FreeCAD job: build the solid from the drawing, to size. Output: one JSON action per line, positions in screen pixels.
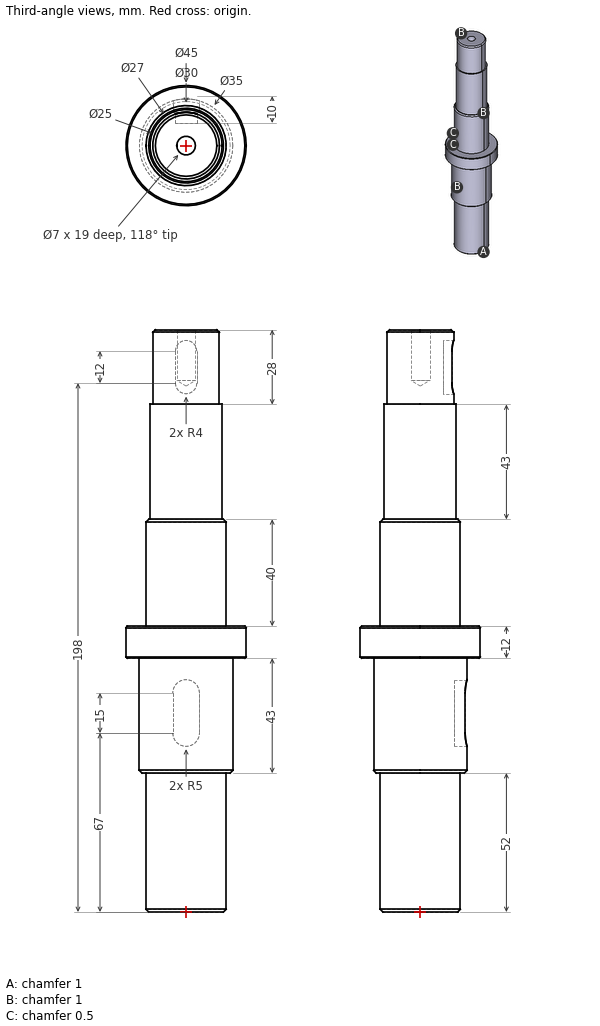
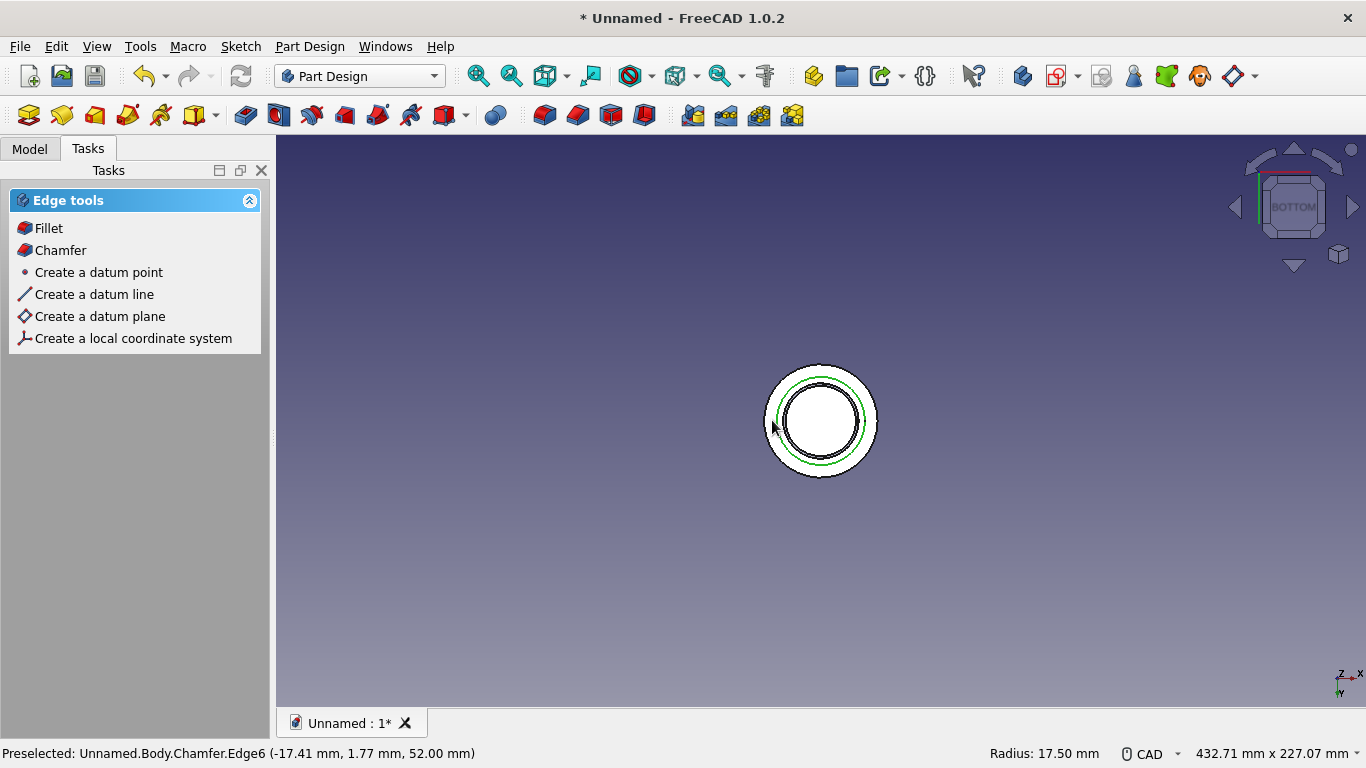
{"action": "key", "text": "0"}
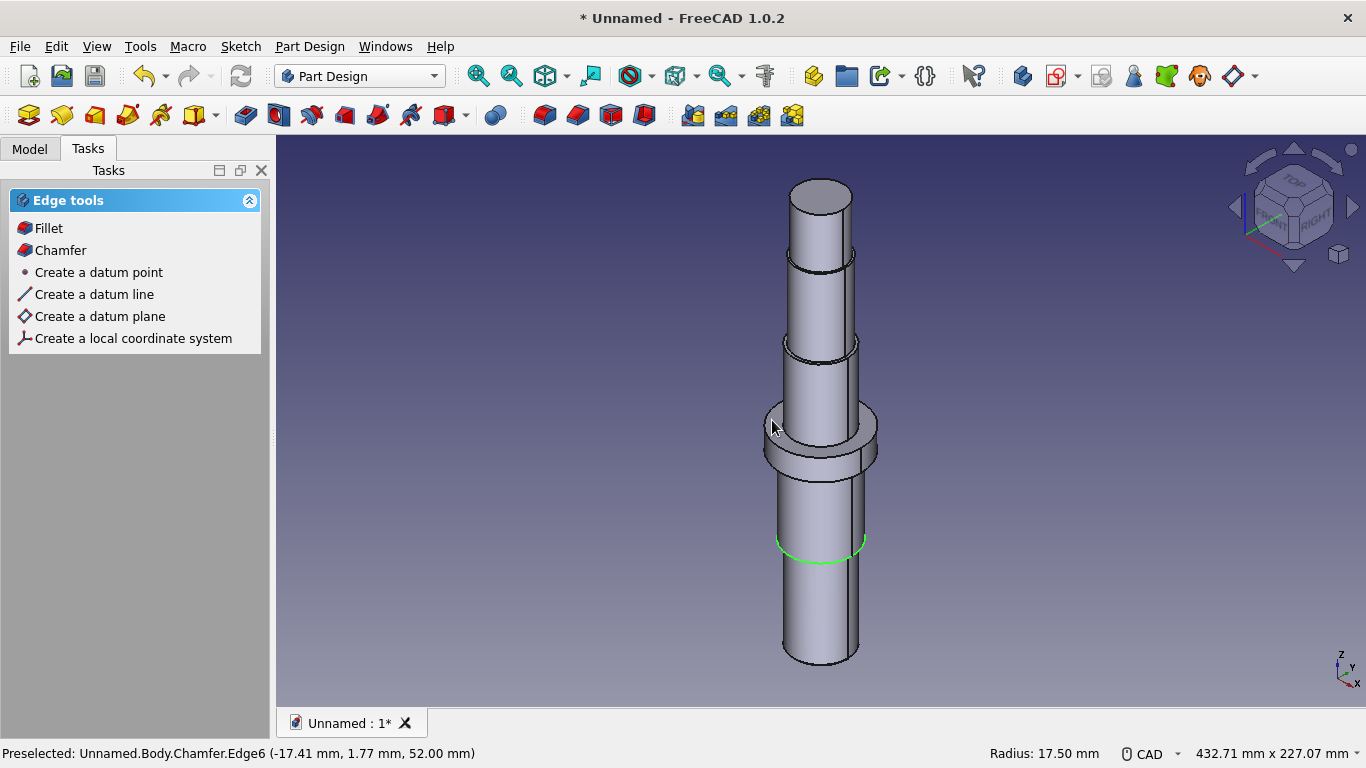
{"action": "left_click", "coordinate": [787, 352], "text": "ctrl"}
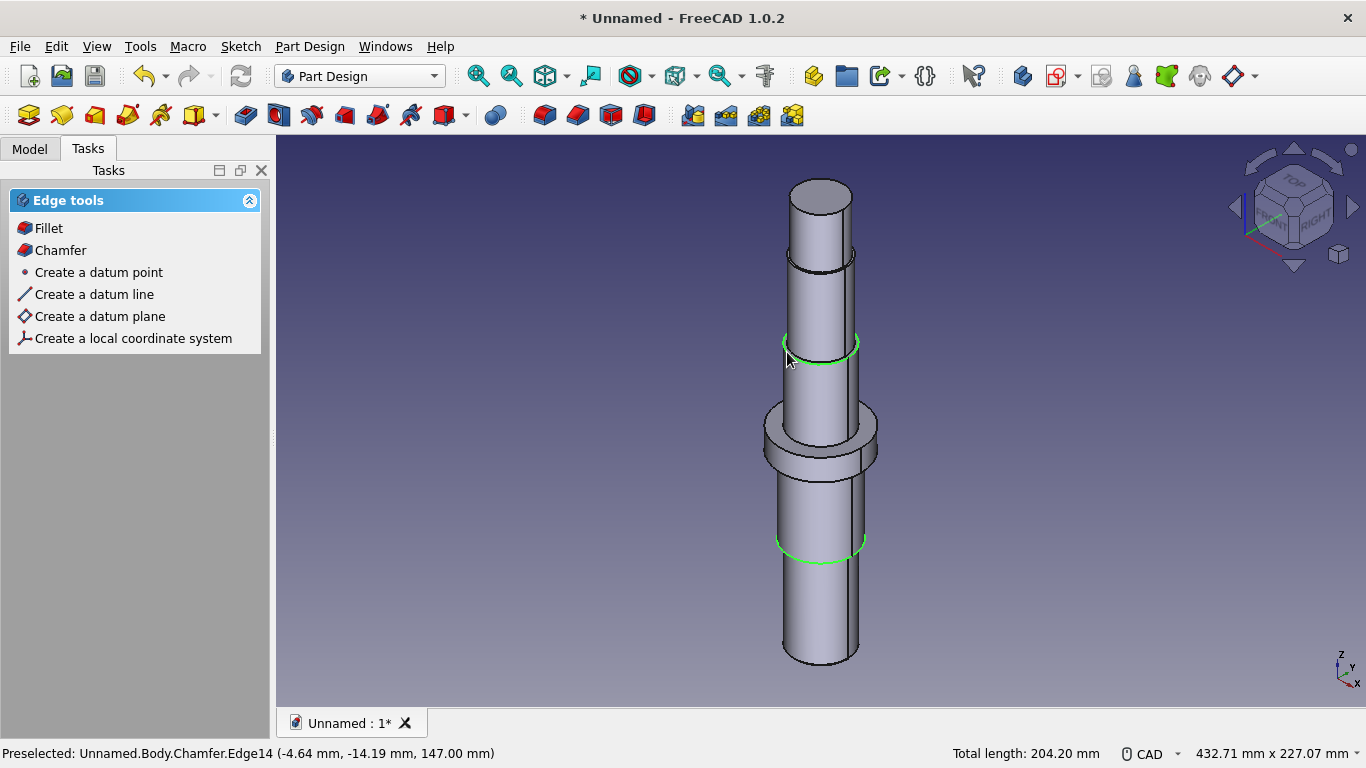
{"action": "left_click", "coordinate": [790, 193], "text": "ctrl"}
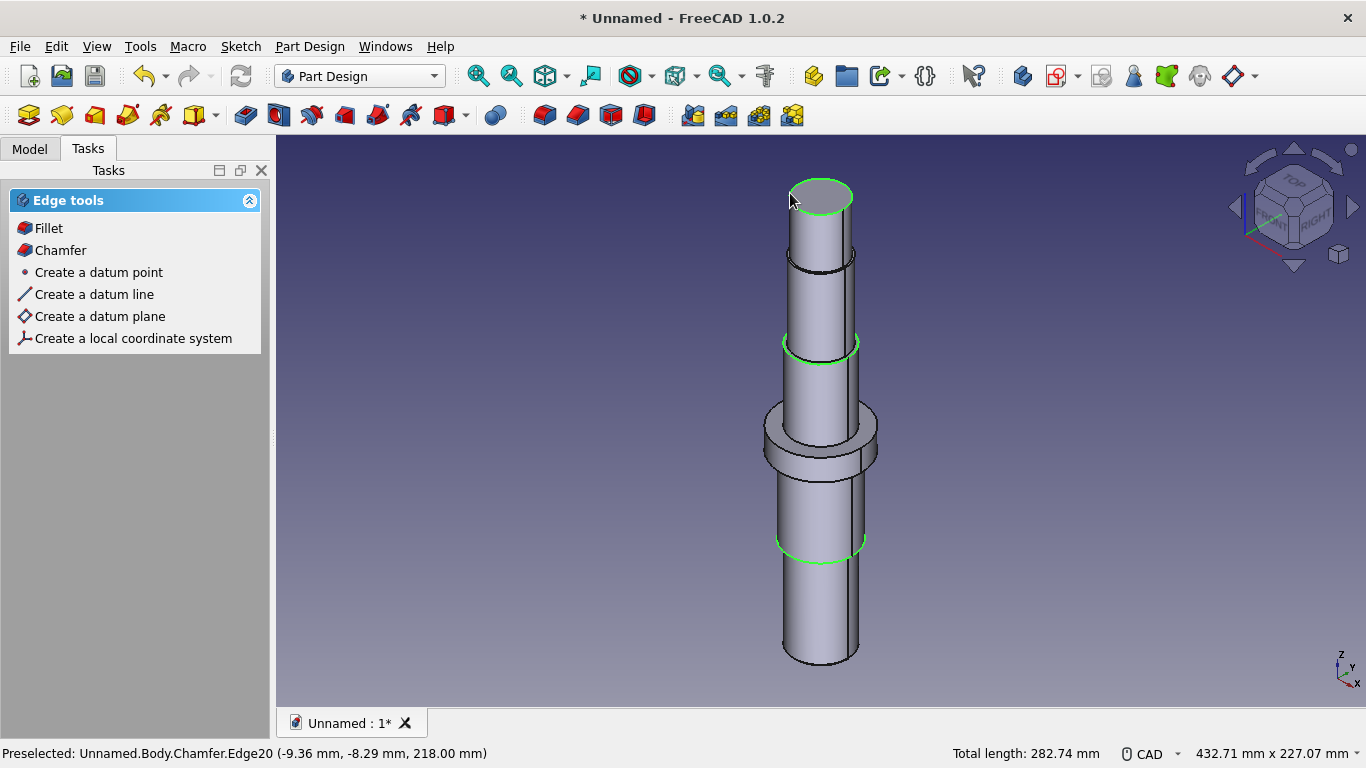
{"action": "left_click", "coordinate": [578, 116]}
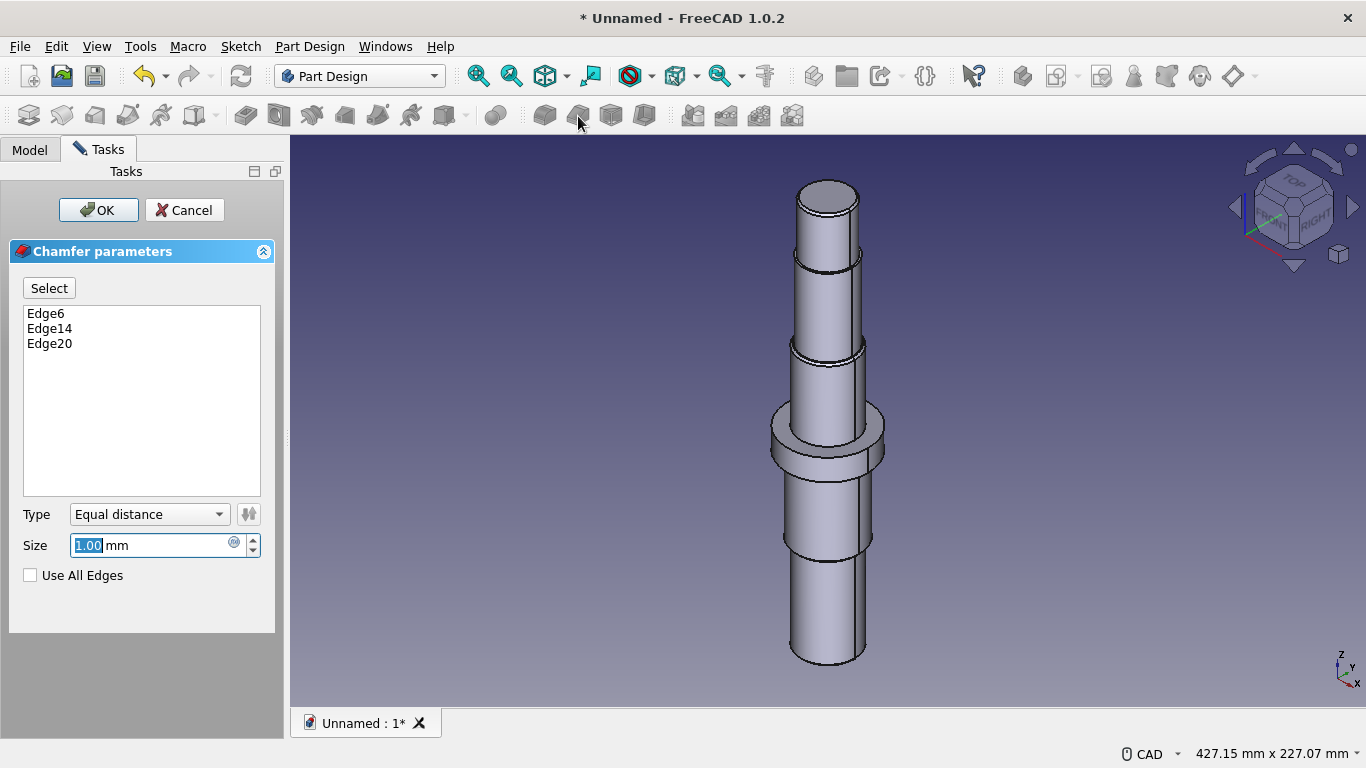
{"action": "type", "text": "1"}
{"action": "key", "text": "Tab"}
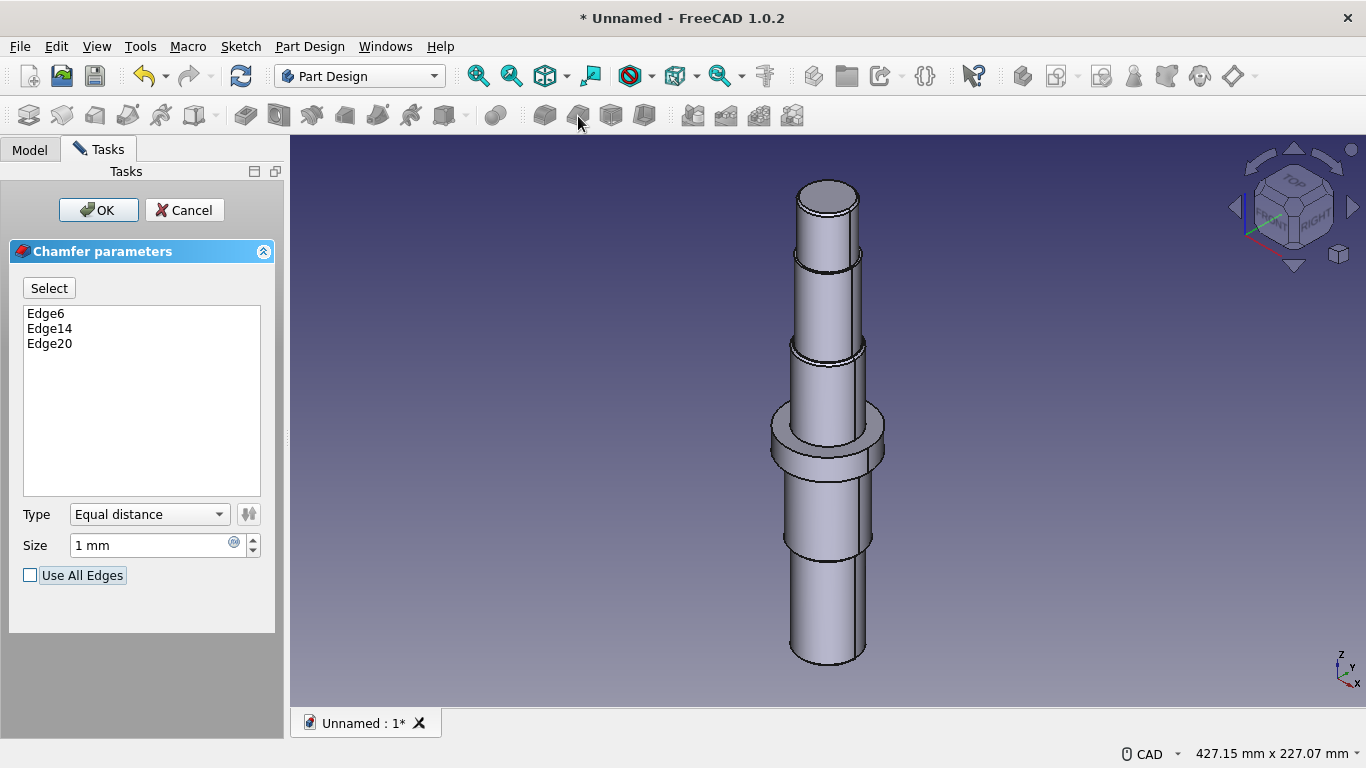
{"action": "left_click", "coordinate": [99, 210]}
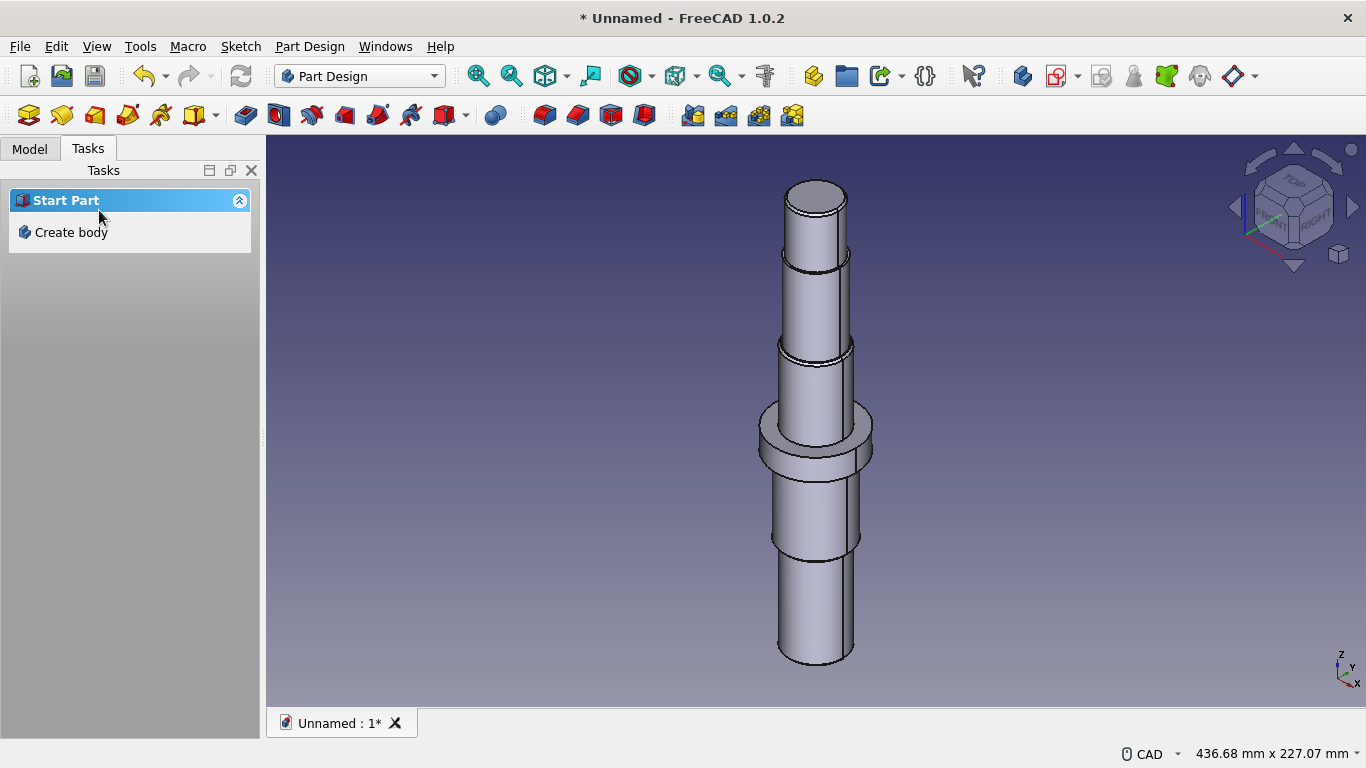
{"action": "left_click", "coordinate": [765, 464]}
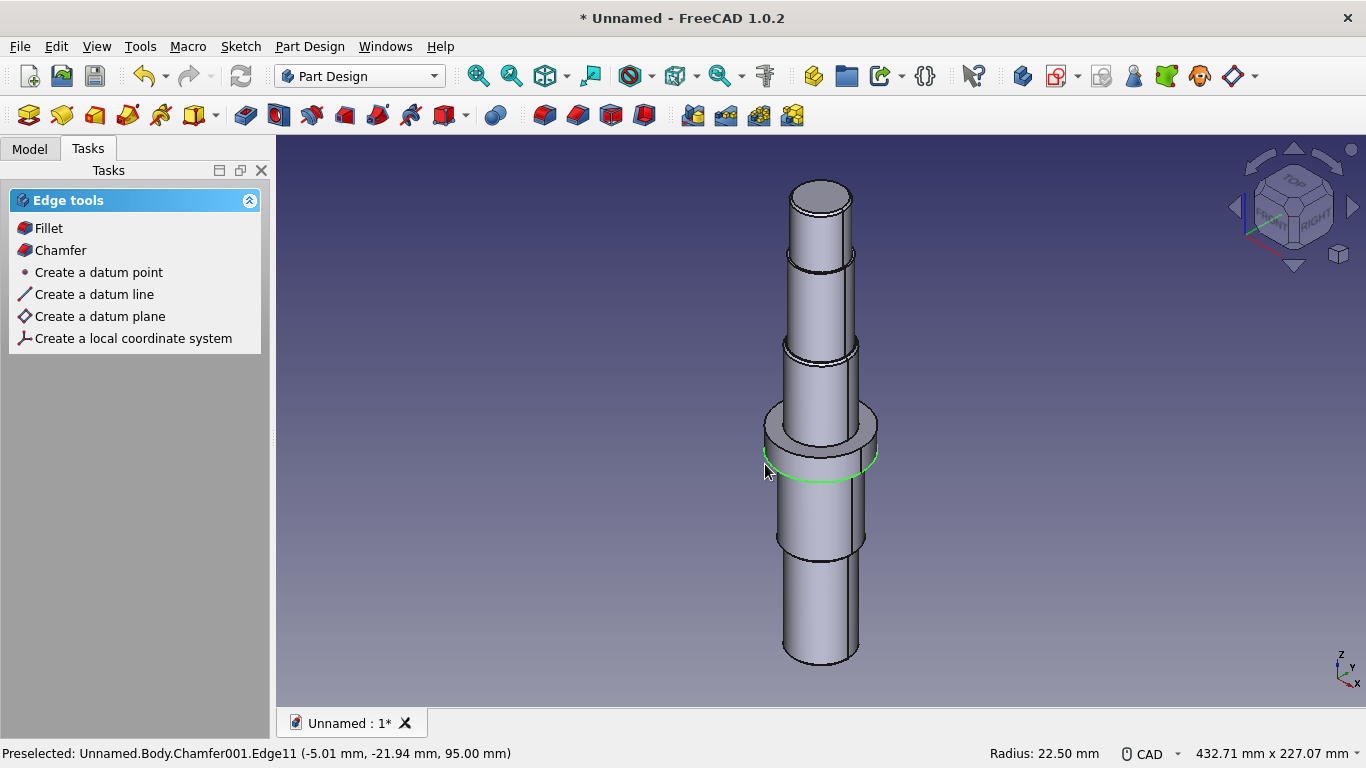
{"action": "left_click", "coordinate": [770, 439], "text": "ctrl"}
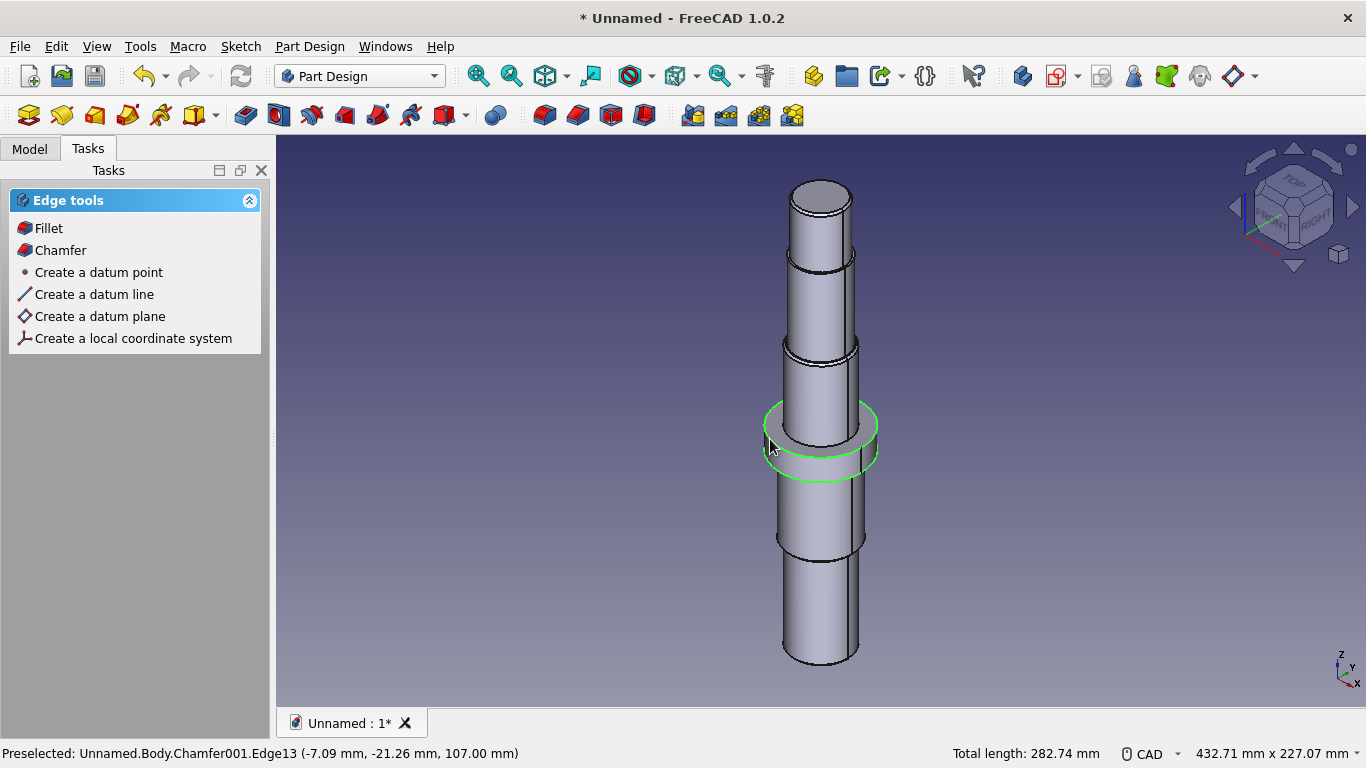
{"action": "left_click", "coordinate": [578, 116]}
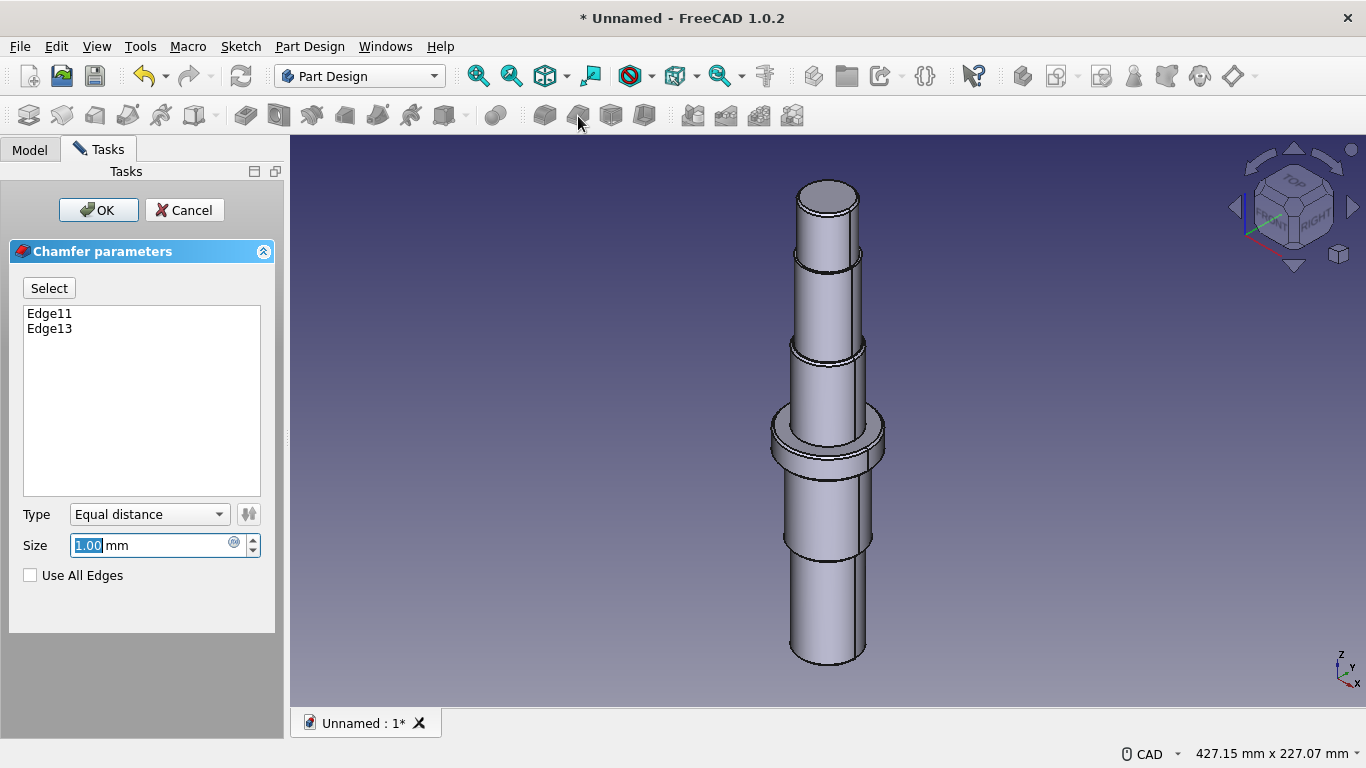
{"action": "type", "text": "0.5"}
{"action": "key", "text": "Tab"}